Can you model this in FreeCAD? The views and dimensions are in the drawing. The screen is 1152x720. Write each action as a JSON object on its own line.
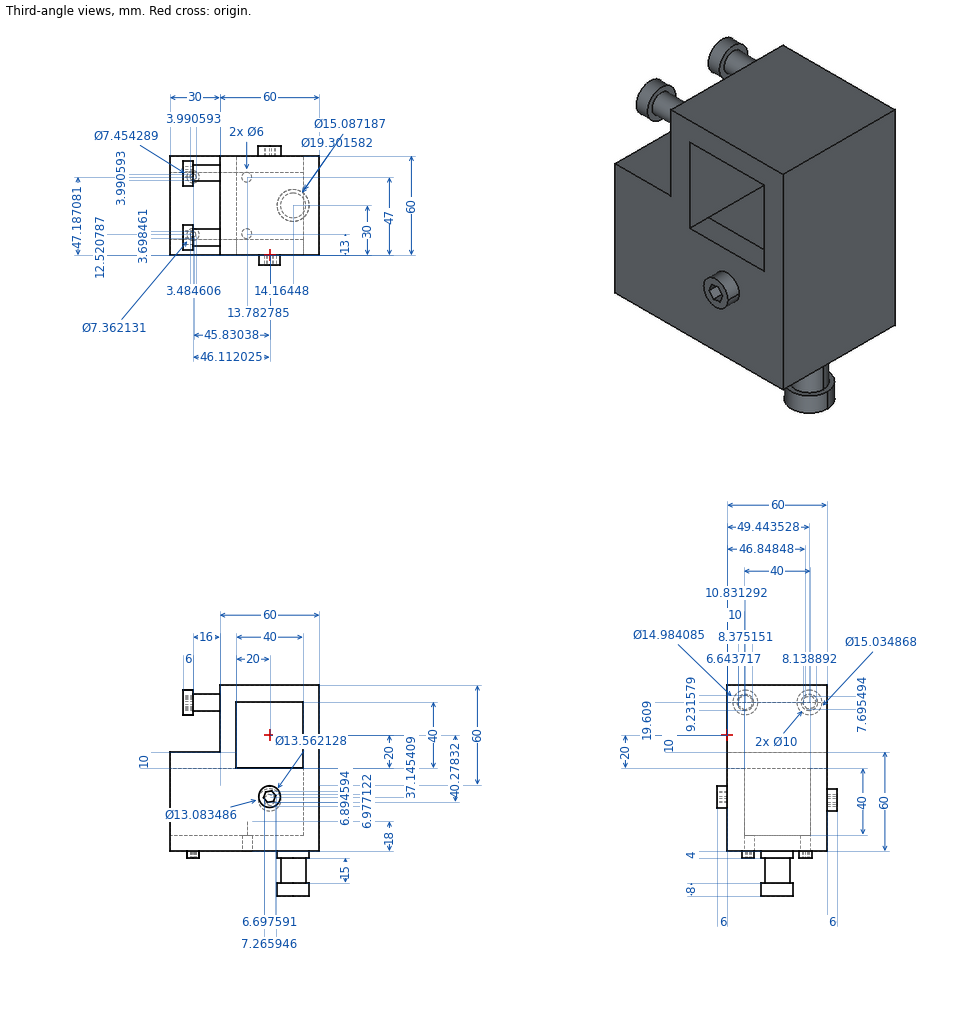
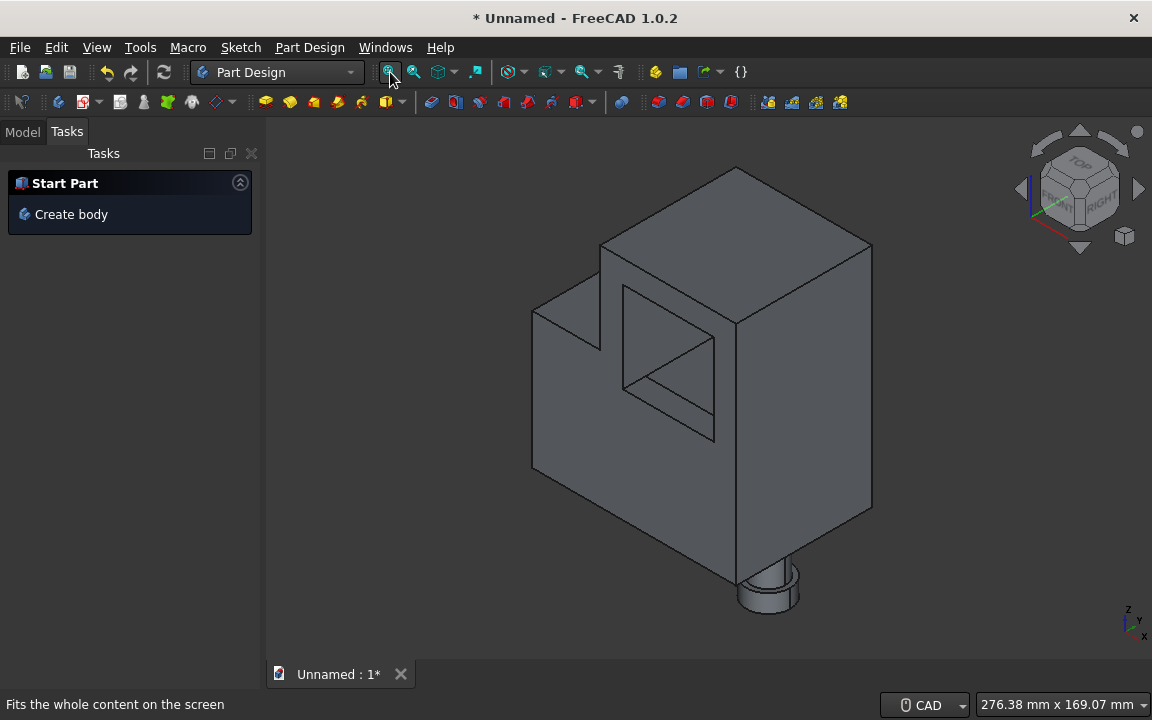
{"action": "left_click", "coordinate": [663, 486]}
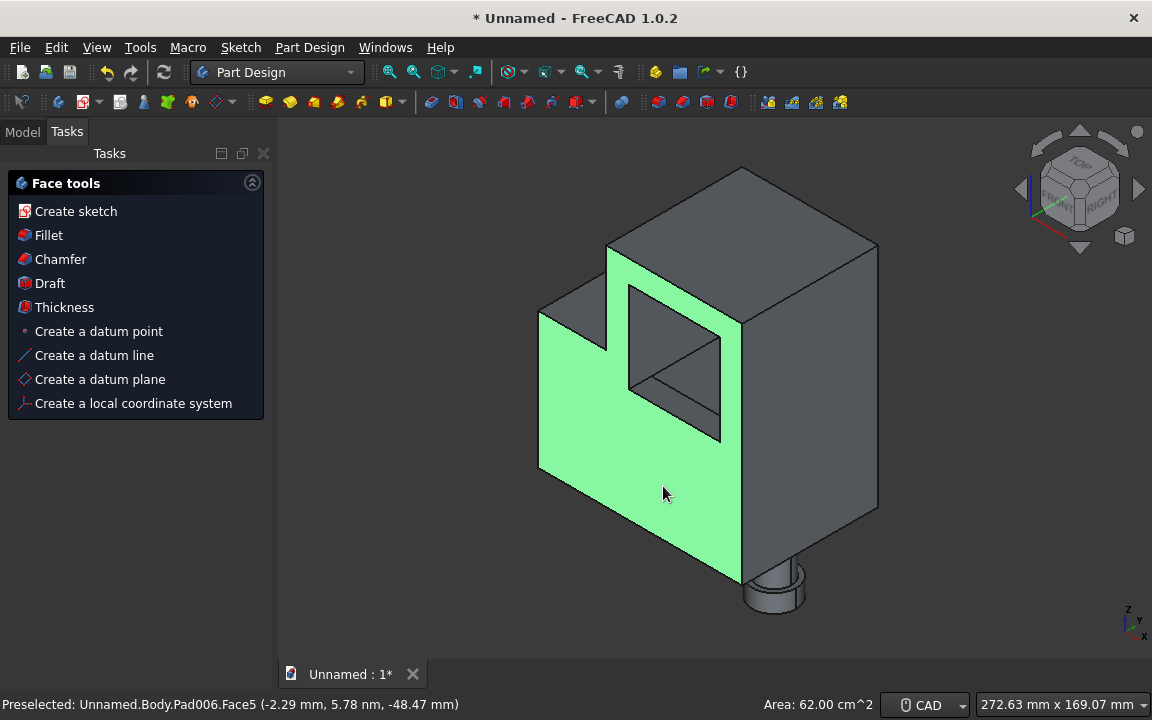
{"action": "left_click", "coordinate": [84, 102]}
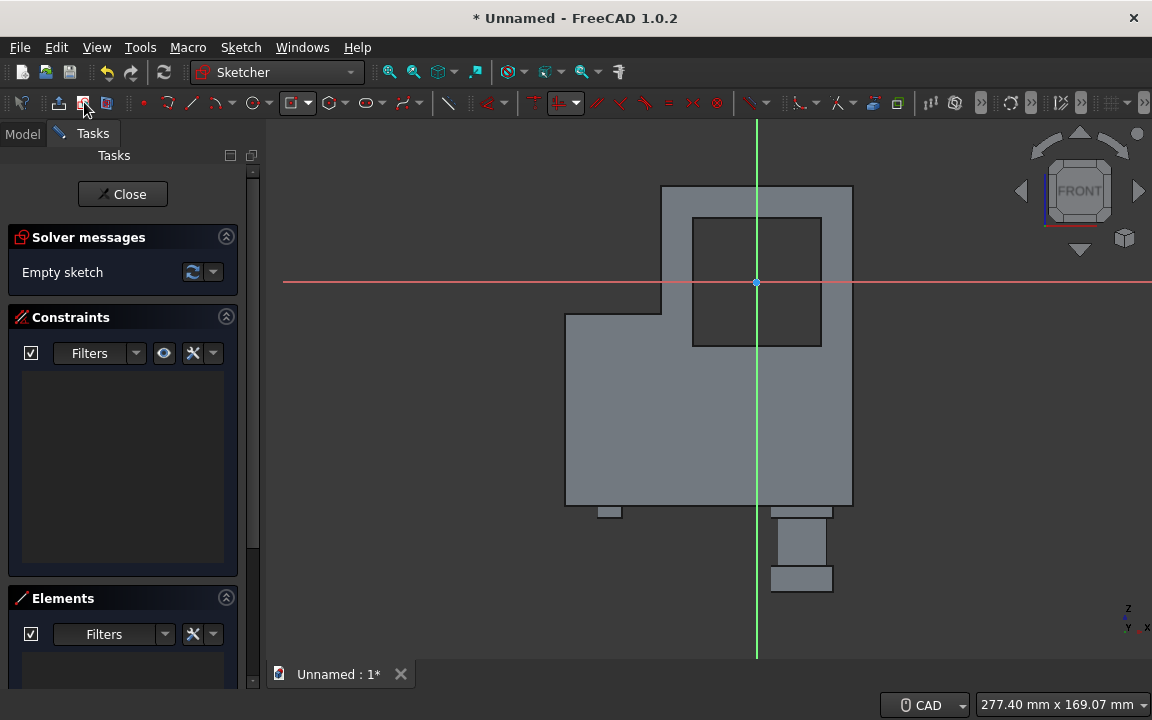
{"action": "scroll", "coordinate": [771, 402], "scroll_direction": "up", "scroll_amount": 11}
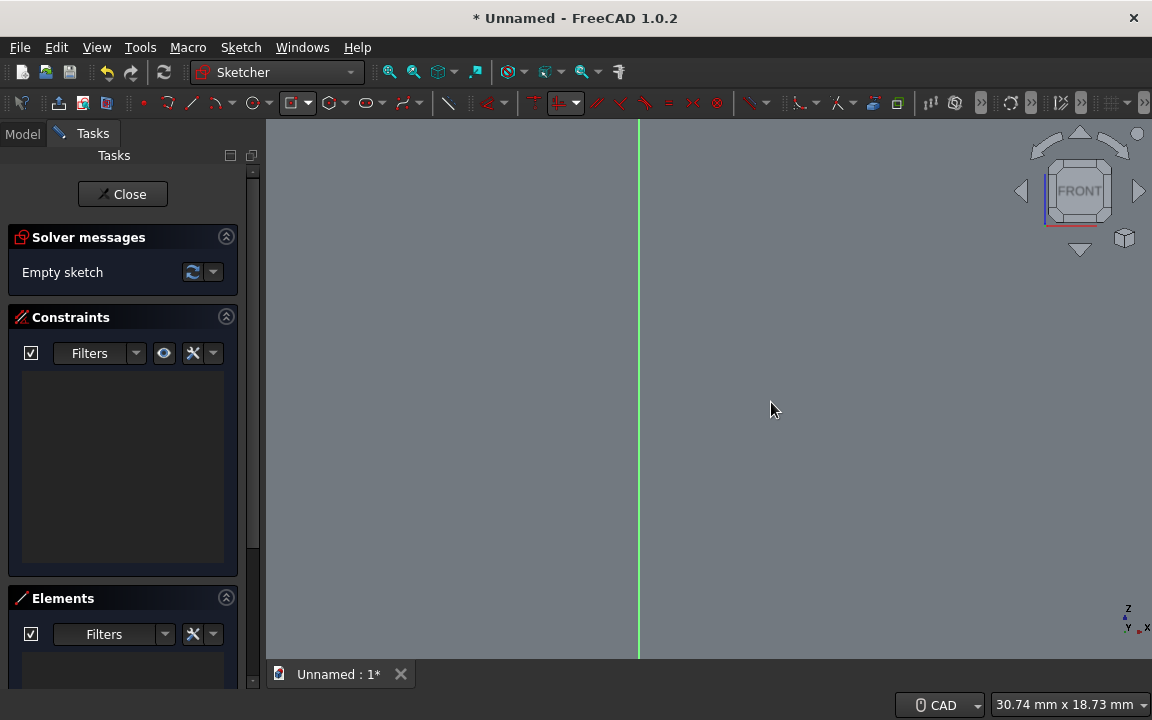
{"action": "left_click", "coordinate": [330, 104]}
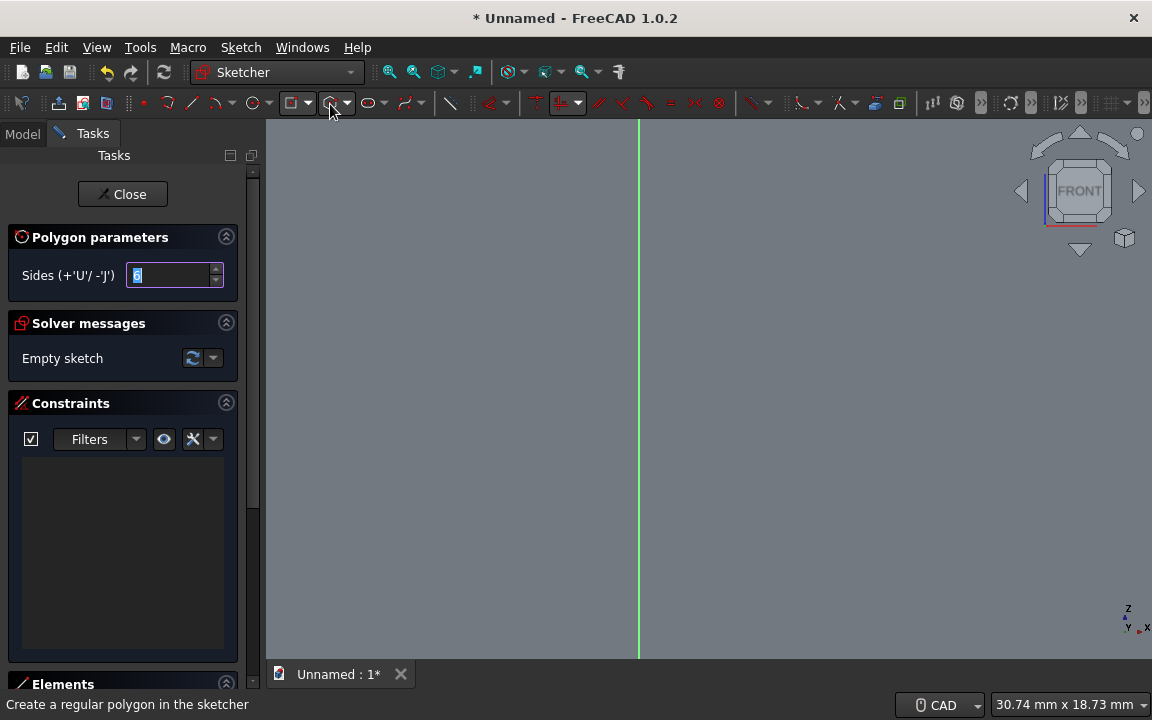
{"action": "left_click", "coordinate": [639, 386]}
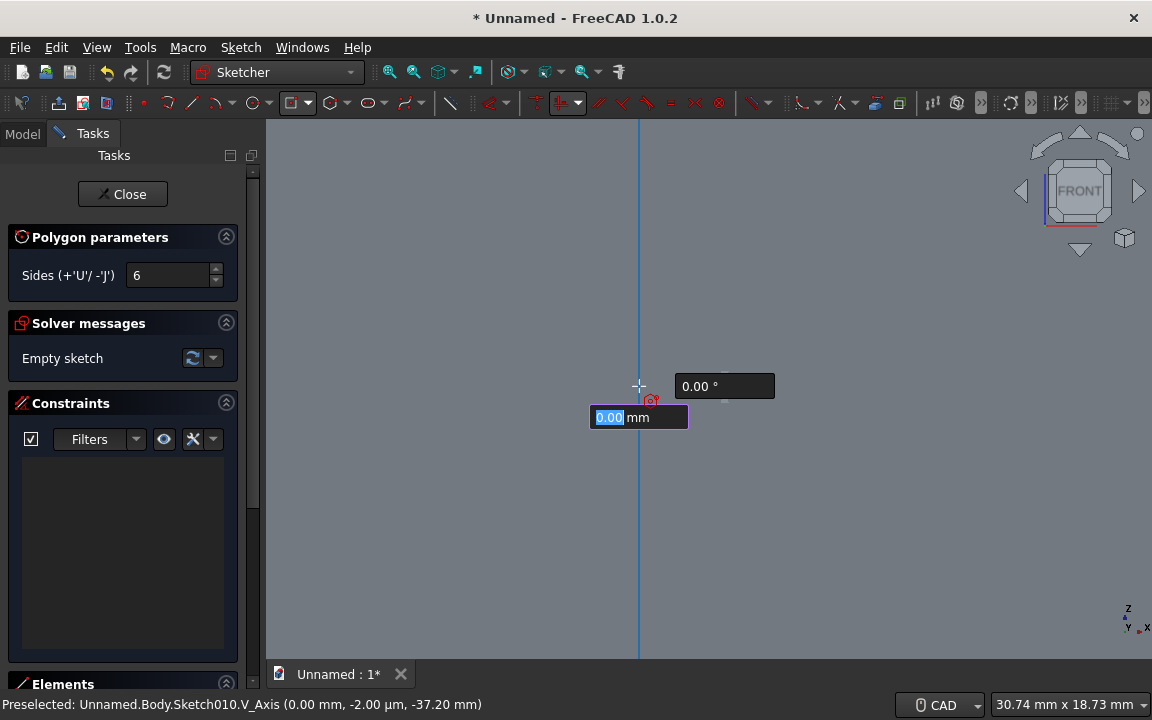
{"action": "left_click", "coordinate": [744, 368]}
{"action": "right_click", "coordinate": [744, 368]}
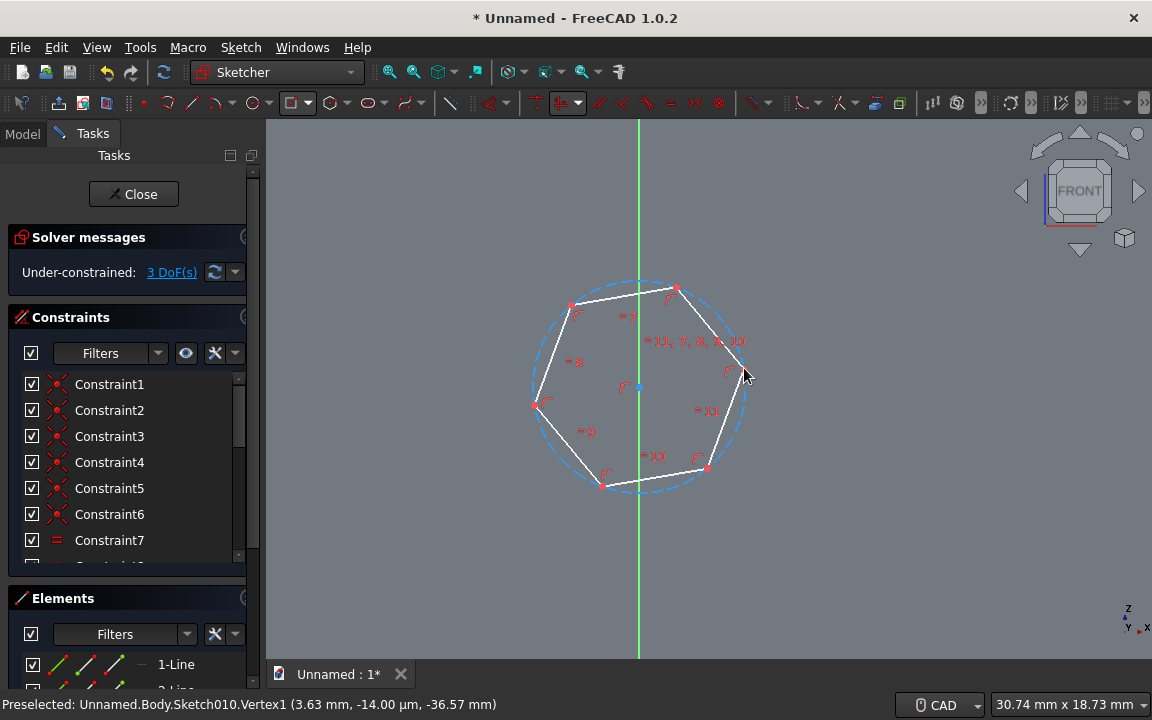
{"action": "left_click", "coordinate": [254, 104]}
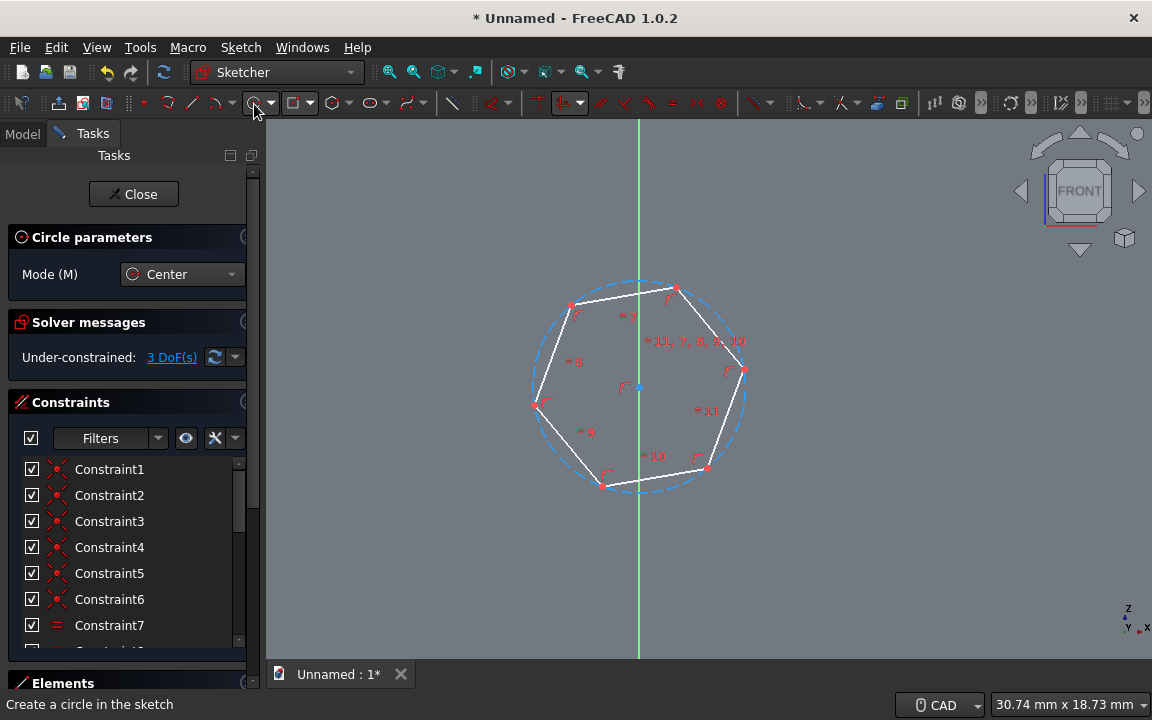
{"action": "left_click", "coordinate": [639, 387]}
{"action": "left_click", "coordinate": [773, 252]}
{"action": "key", "text": "Escape"}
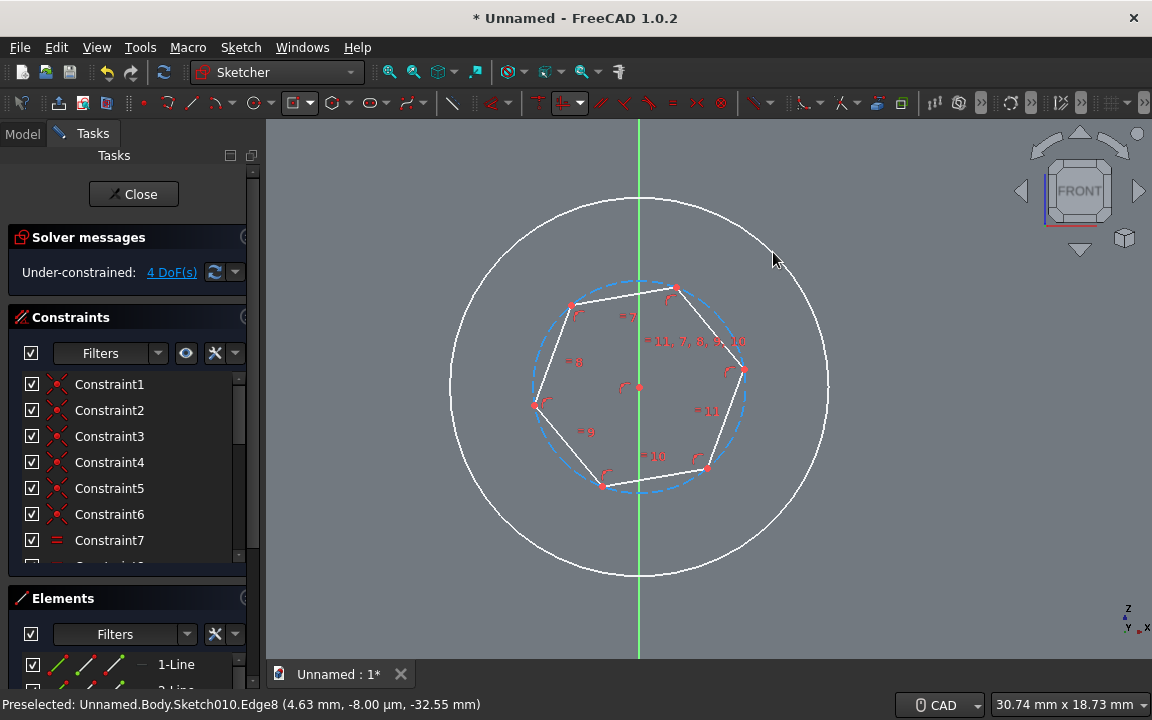
{"action": "left_click", "coordinate": [492, 104]}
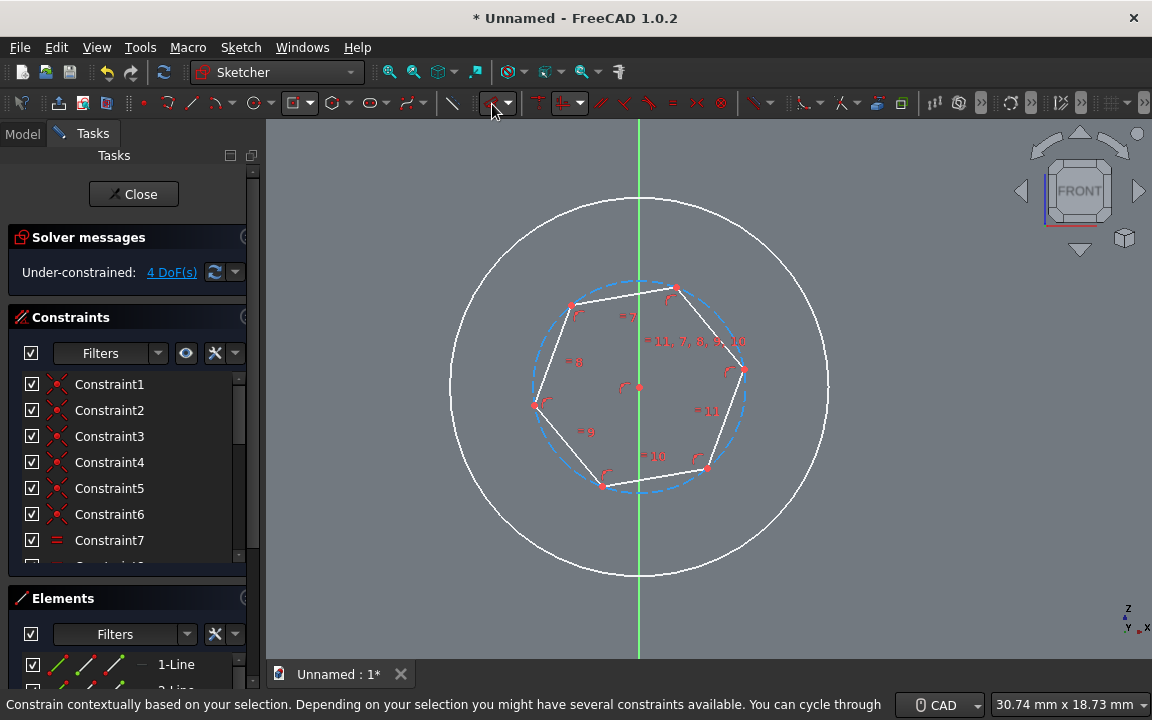
{"action": "left_click", "coordinate": [773, 253]}
{"action": "left_click", "coordinate": [796, 230]}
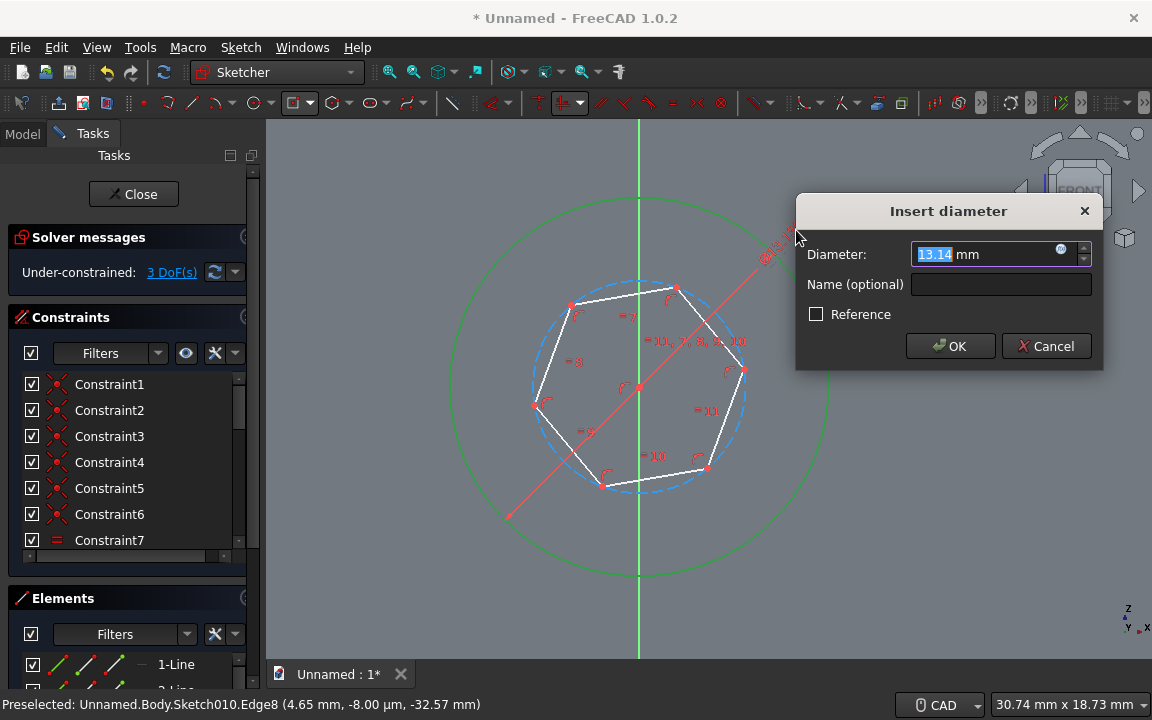
{"action": "type", "text": "13.083486"}
{"action": "key", "text": "Return"}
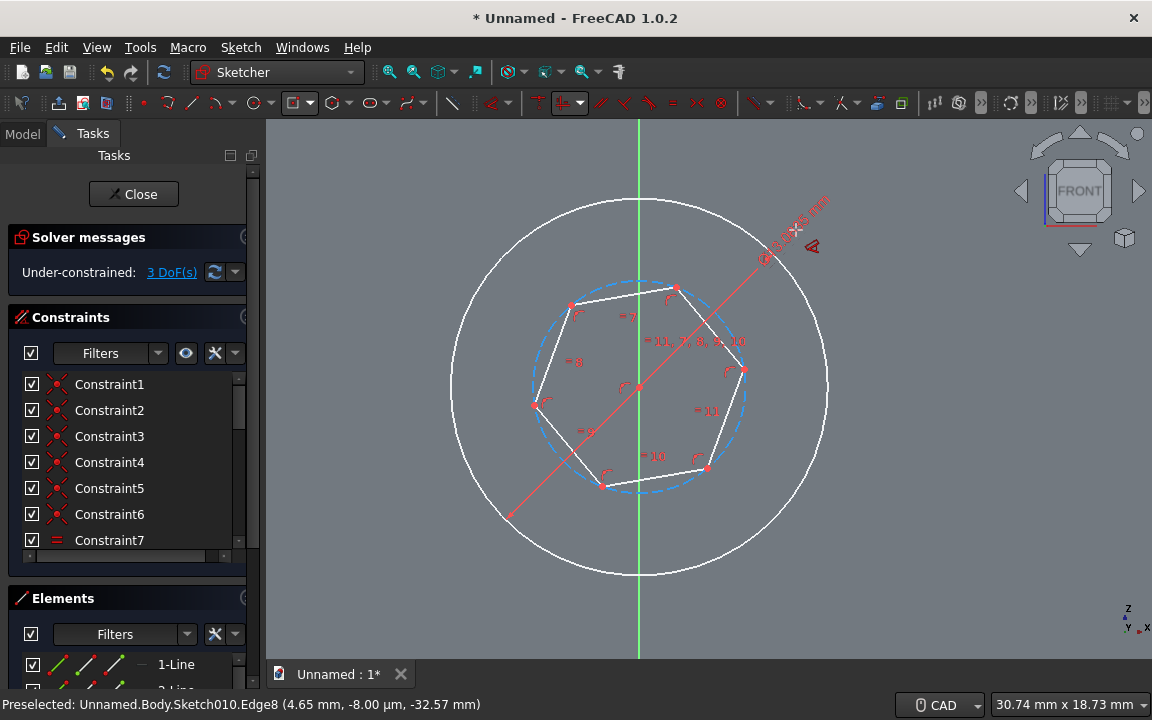
{"action": "left_click", "coordinate": [534, 405]}